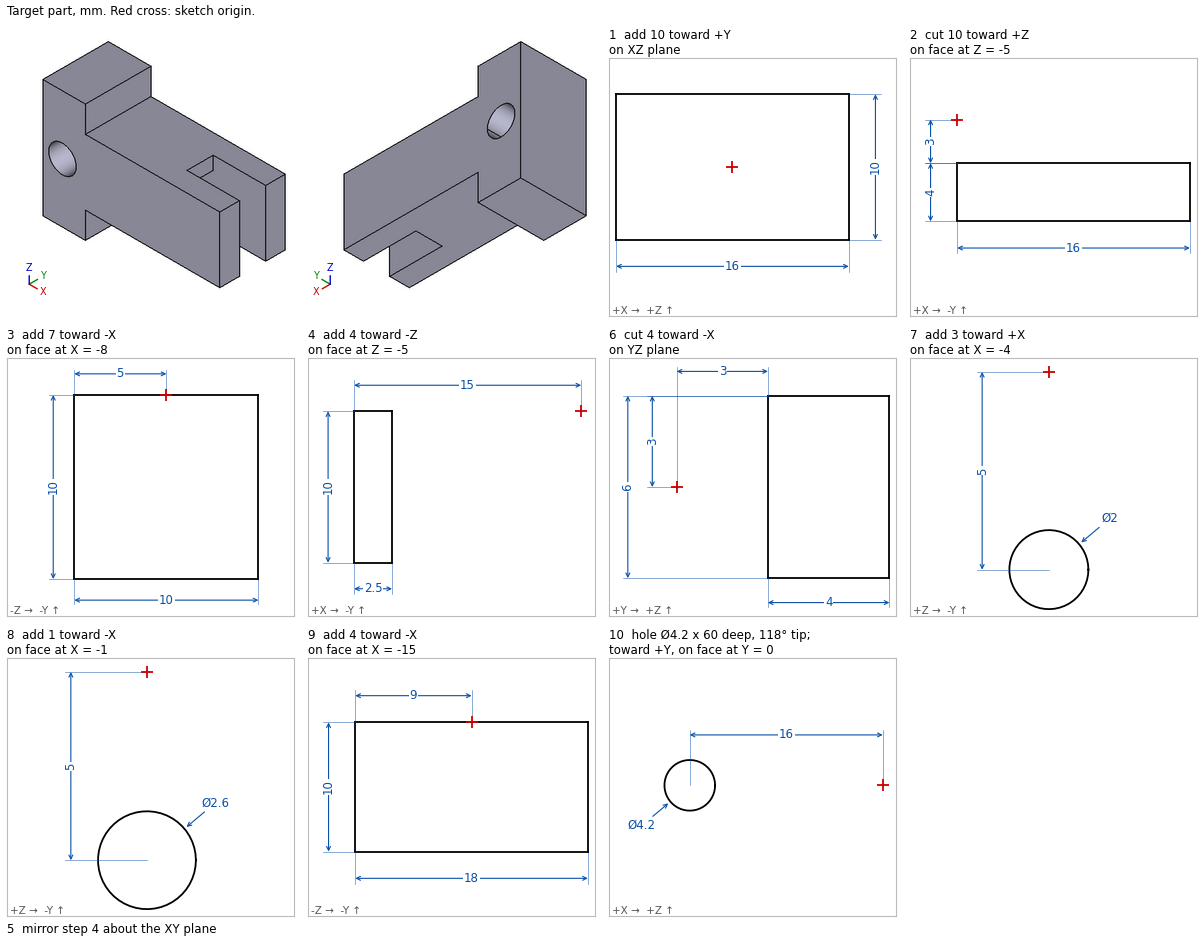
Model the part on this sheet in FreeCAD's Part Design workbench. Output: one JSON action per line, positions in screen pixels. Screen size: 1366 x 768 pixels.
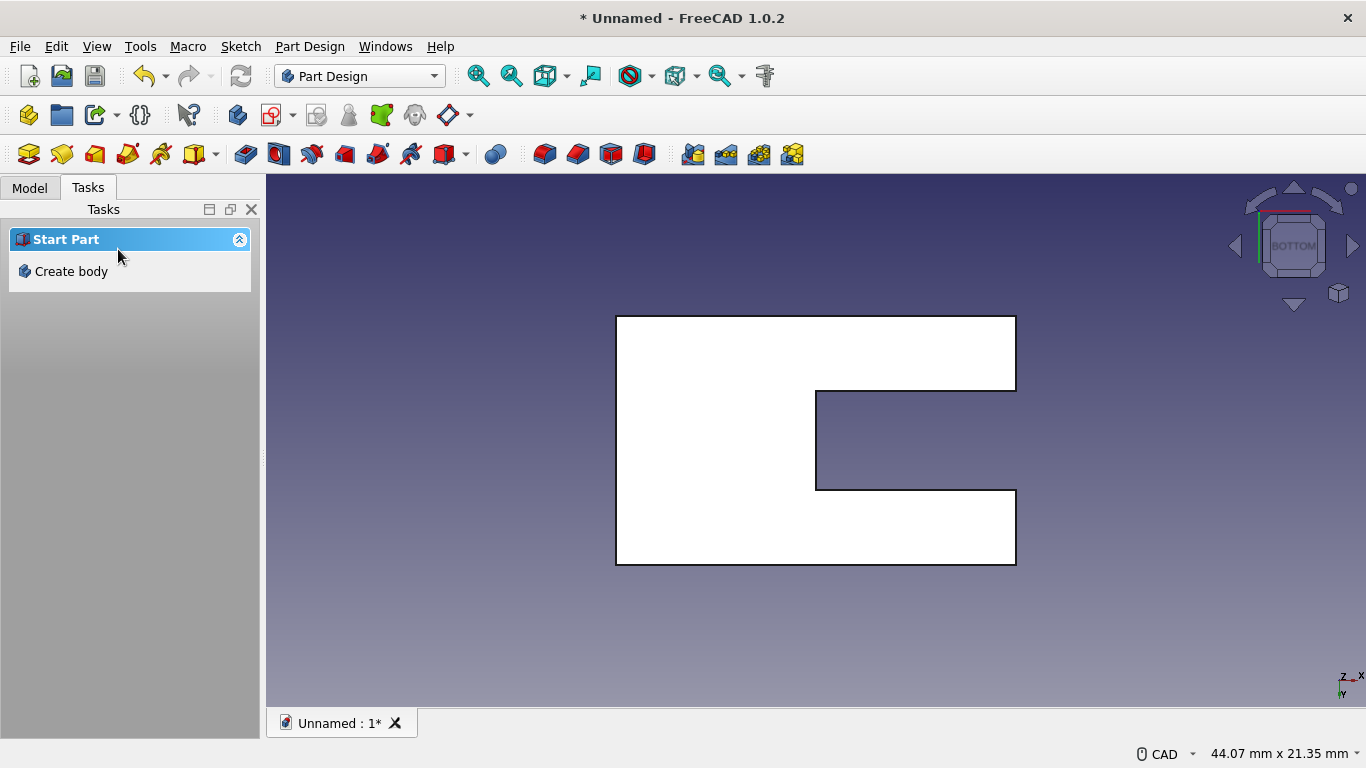
{"action": "key", "text": "6"}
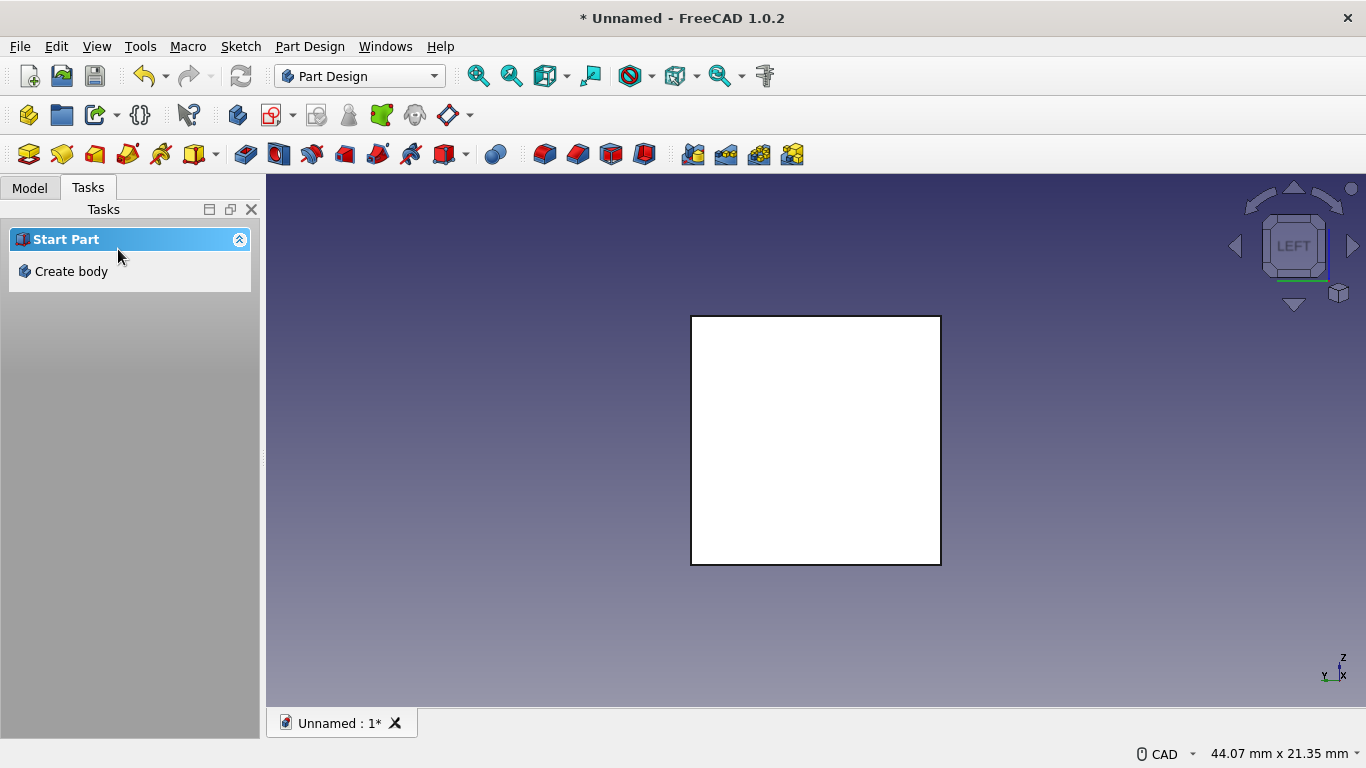
{"action": "left_click", "coordinate": [816, 440]}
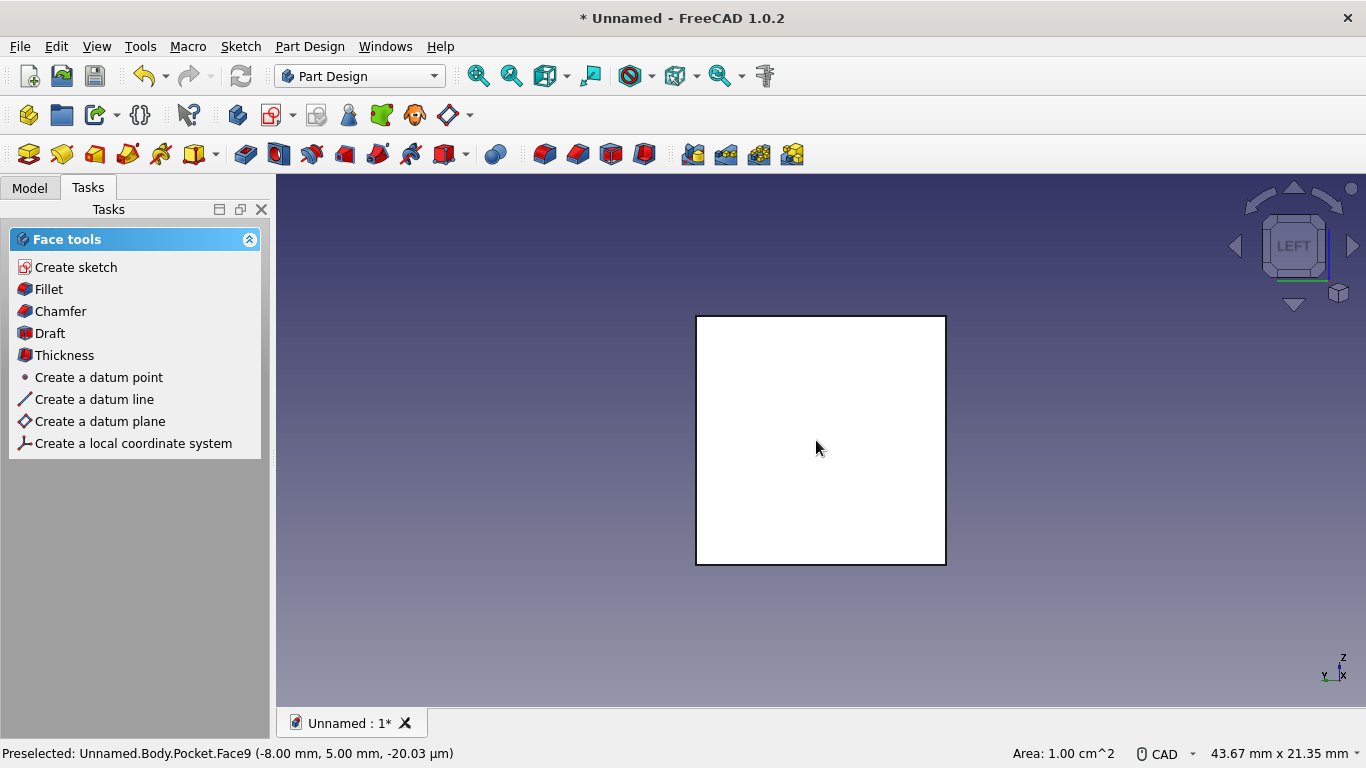
{"action": "left_click", "coordinate": [270, 116]}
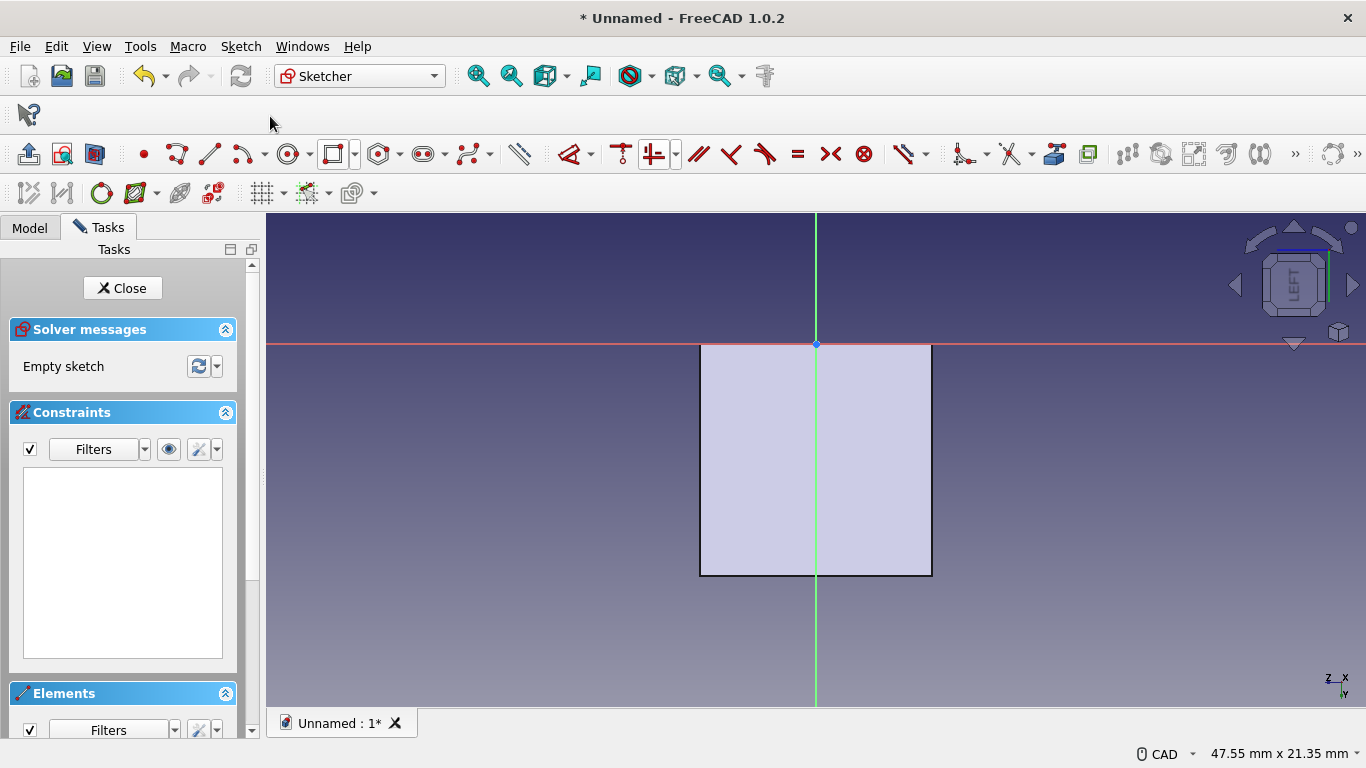
{"action": "left_click", "coordinate": [332, 154]}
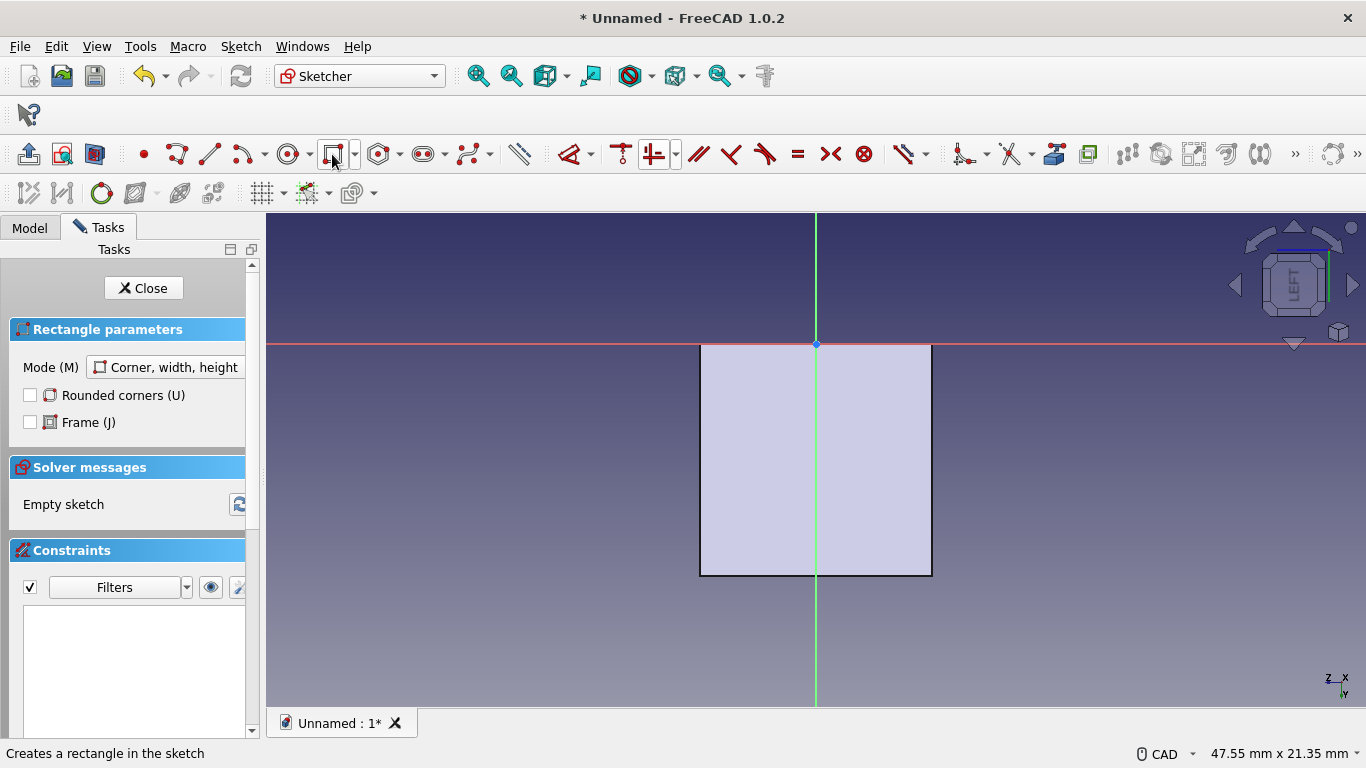
{"action": "left_click", "coordinate": [700, 344]}
{"action": "left_click", "coordinate": [932, 576]}
{"action": "key", "text": "Escape"}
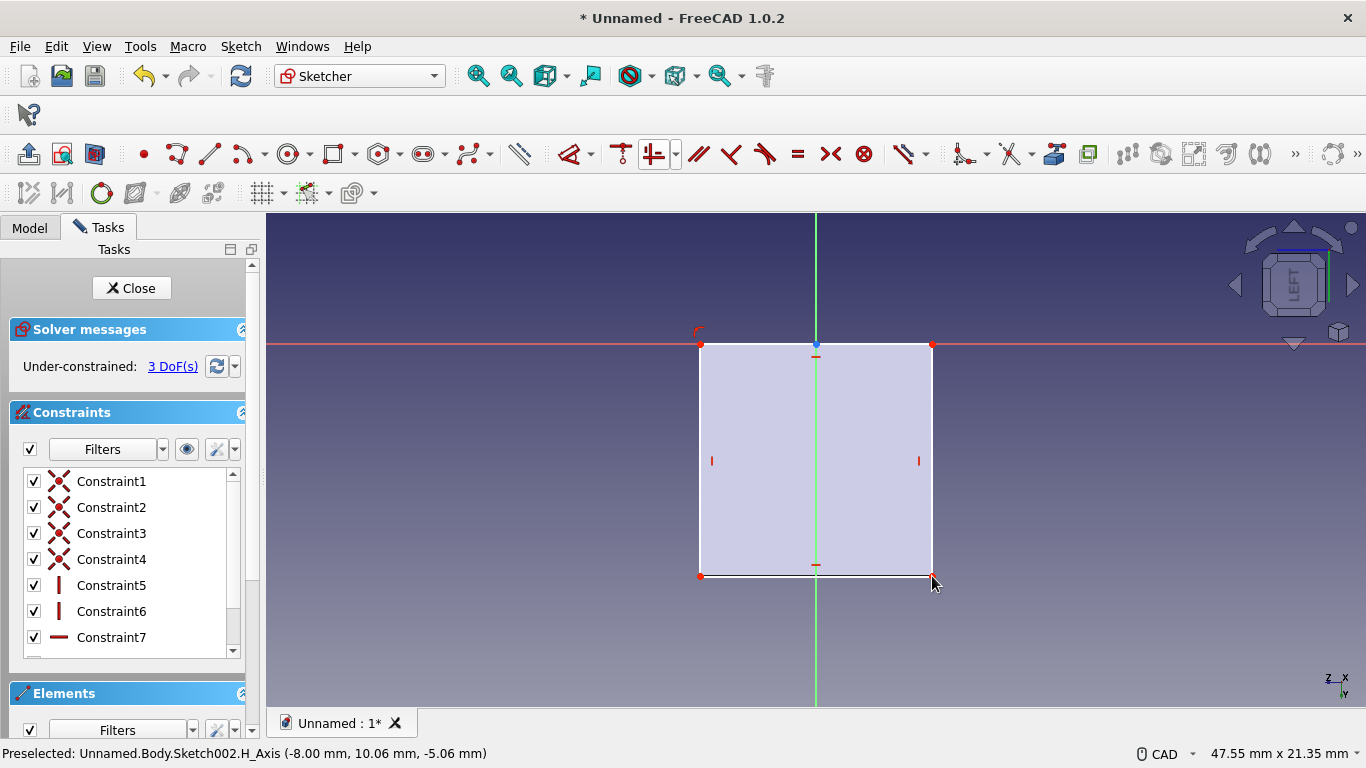
{"action": "left_click", "coordinate": [568, 154]}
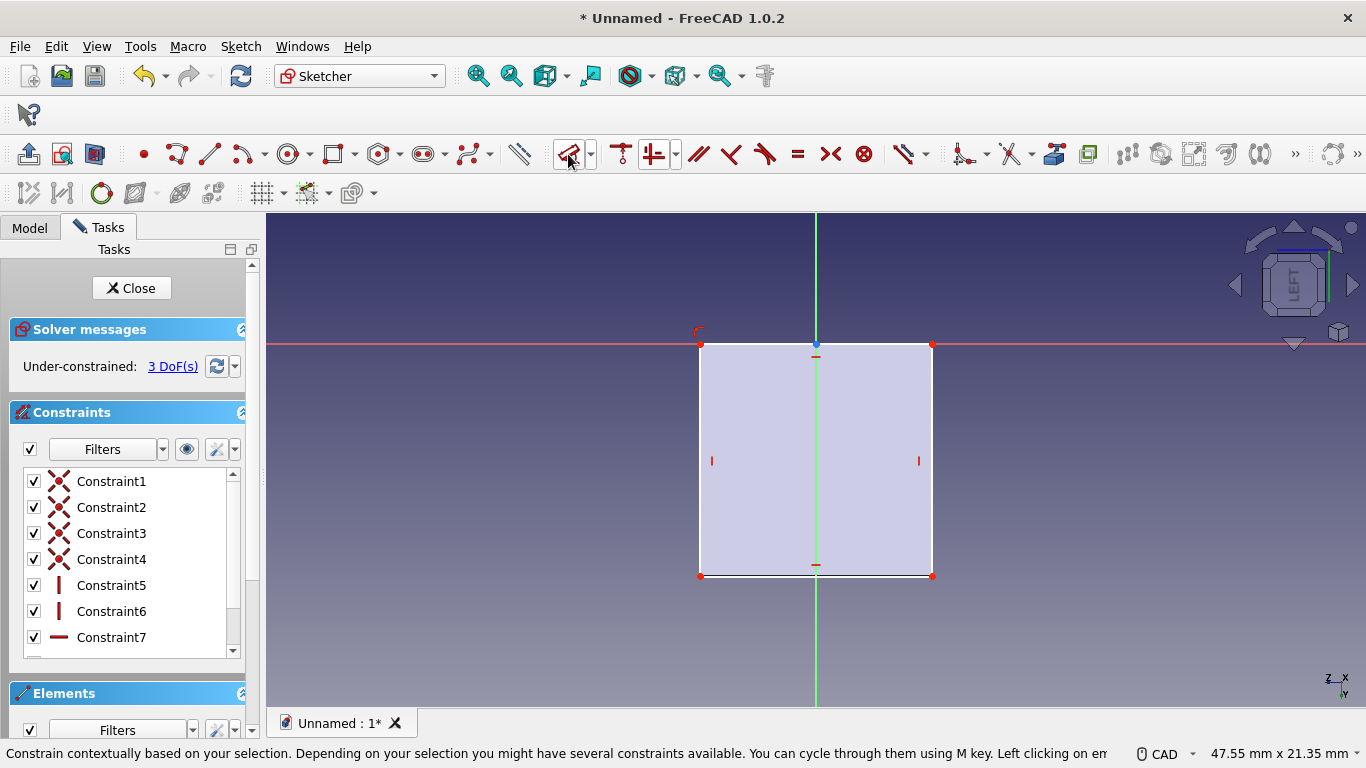
{"action": "left_click", "coordinate": [700, 414]}
{"action": "left_click", "coordinate": [666, 461]}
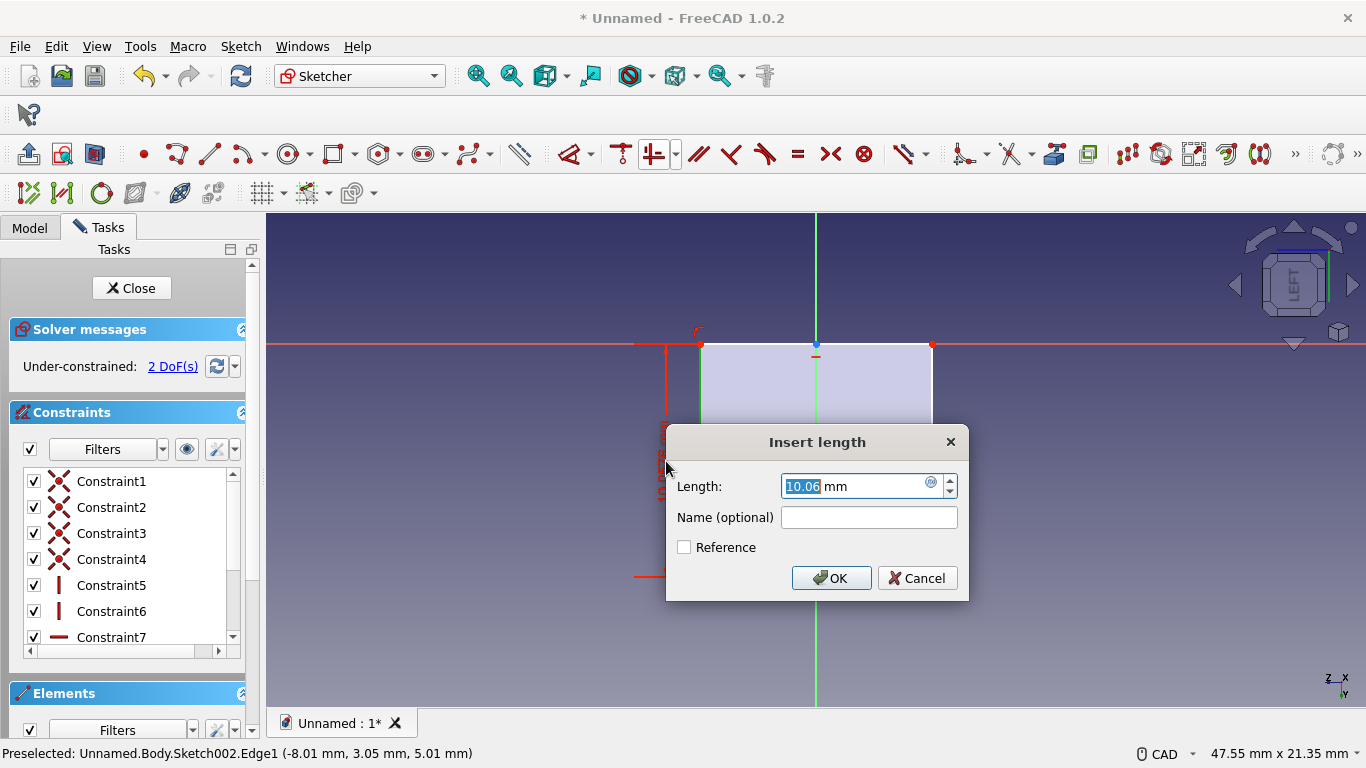
{"action": "type", "text": "10"}
{"action": "key", "text": "Return"}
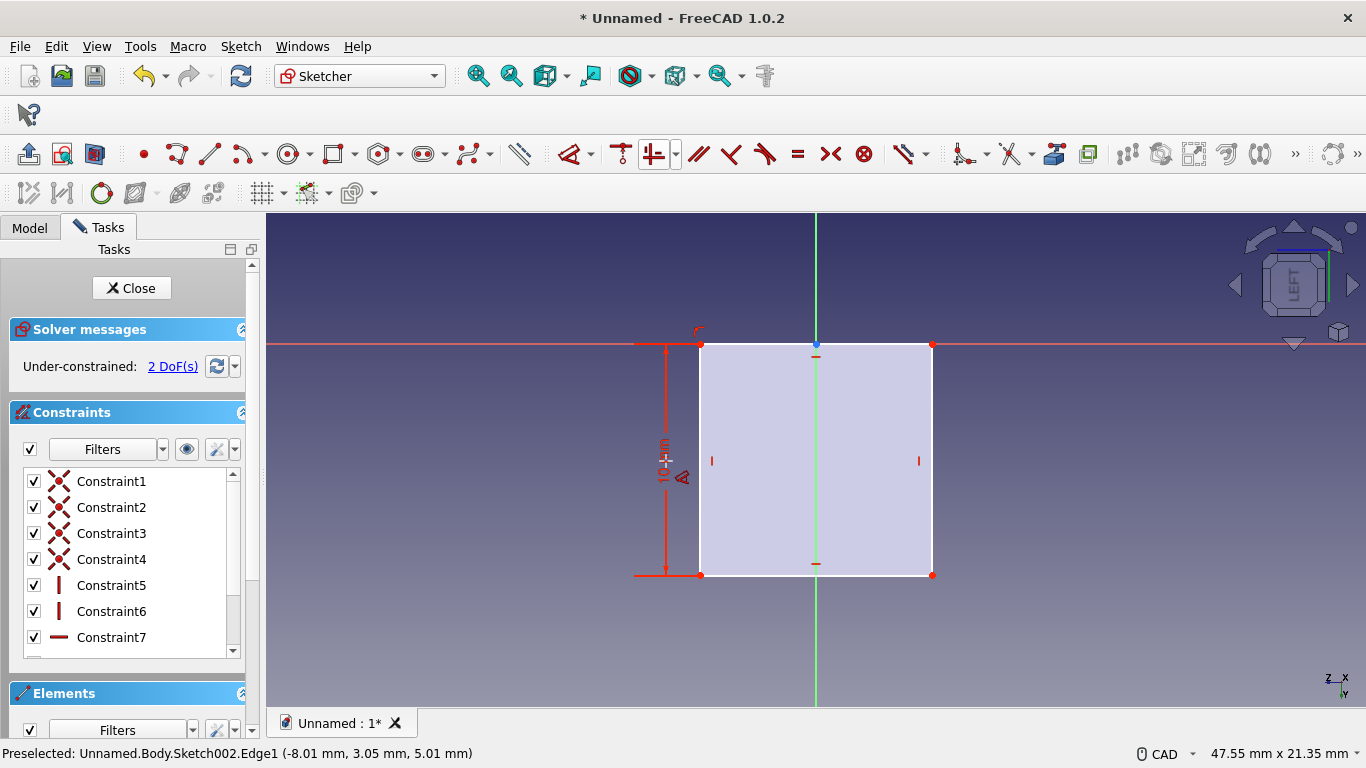
{"action": "left_click", "coordinate": [770, 576]}
{"action": "left_click", "coordinate": [763, 610]}